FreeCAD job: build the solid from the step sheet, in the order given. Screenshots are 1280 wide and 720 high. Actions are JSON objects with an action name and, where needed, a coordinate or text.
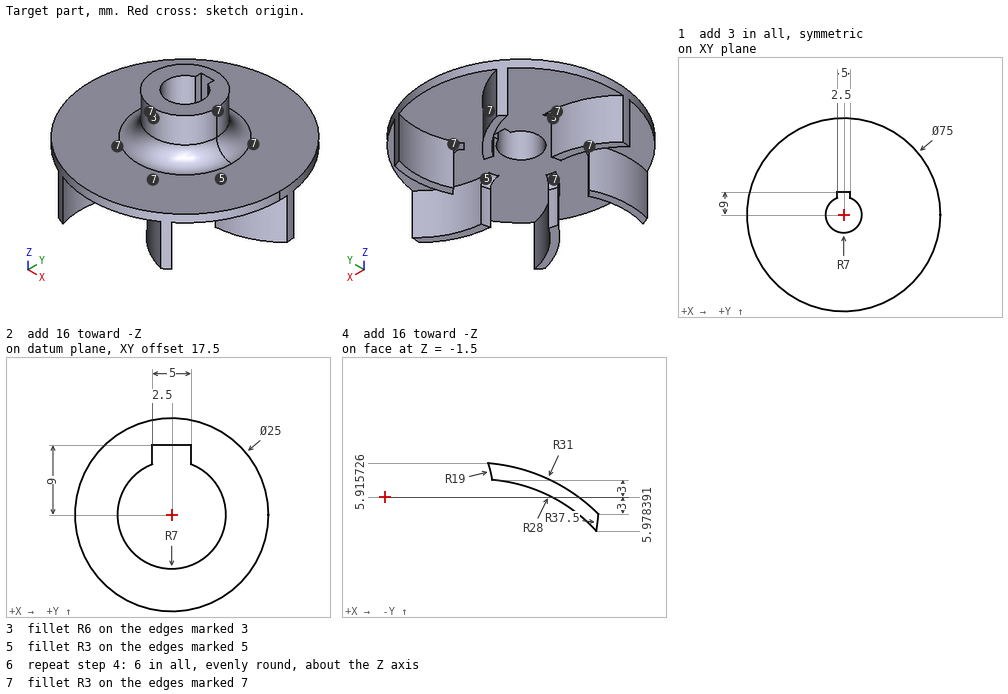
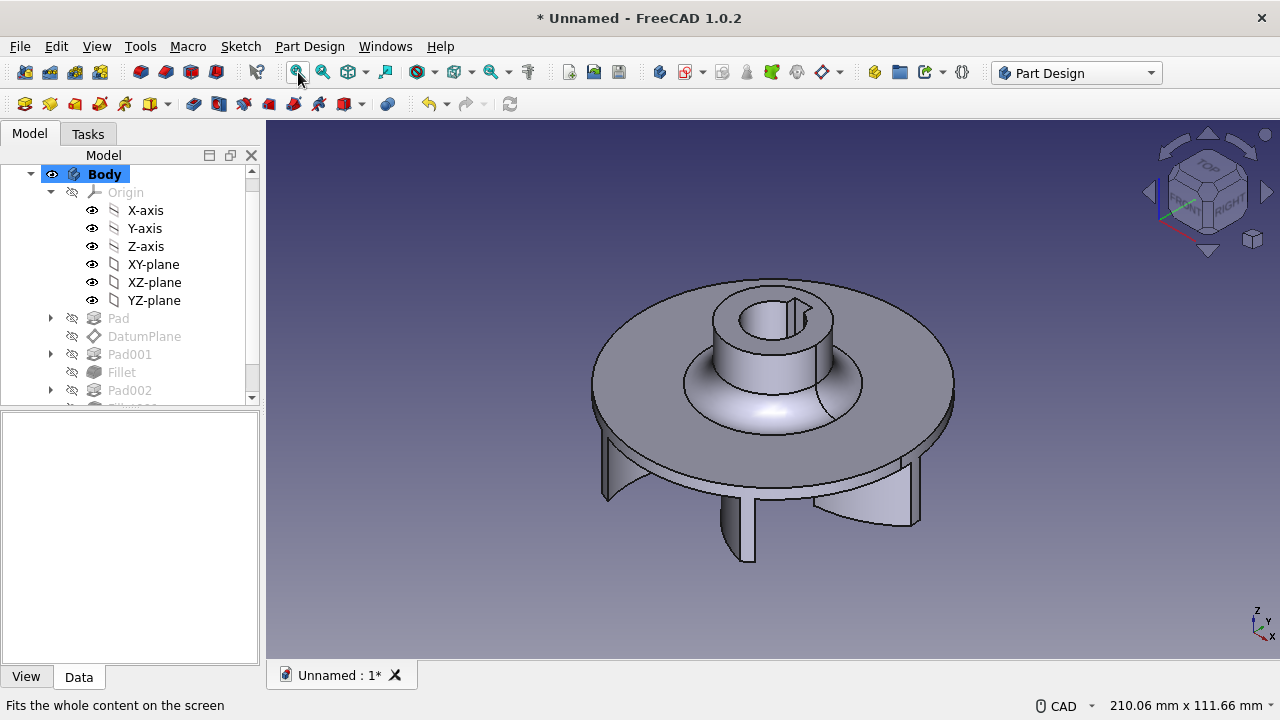
{"action": "scroll", "coordinate": [865, 393], "scroll_direction": "up", "scroll_amount": 6}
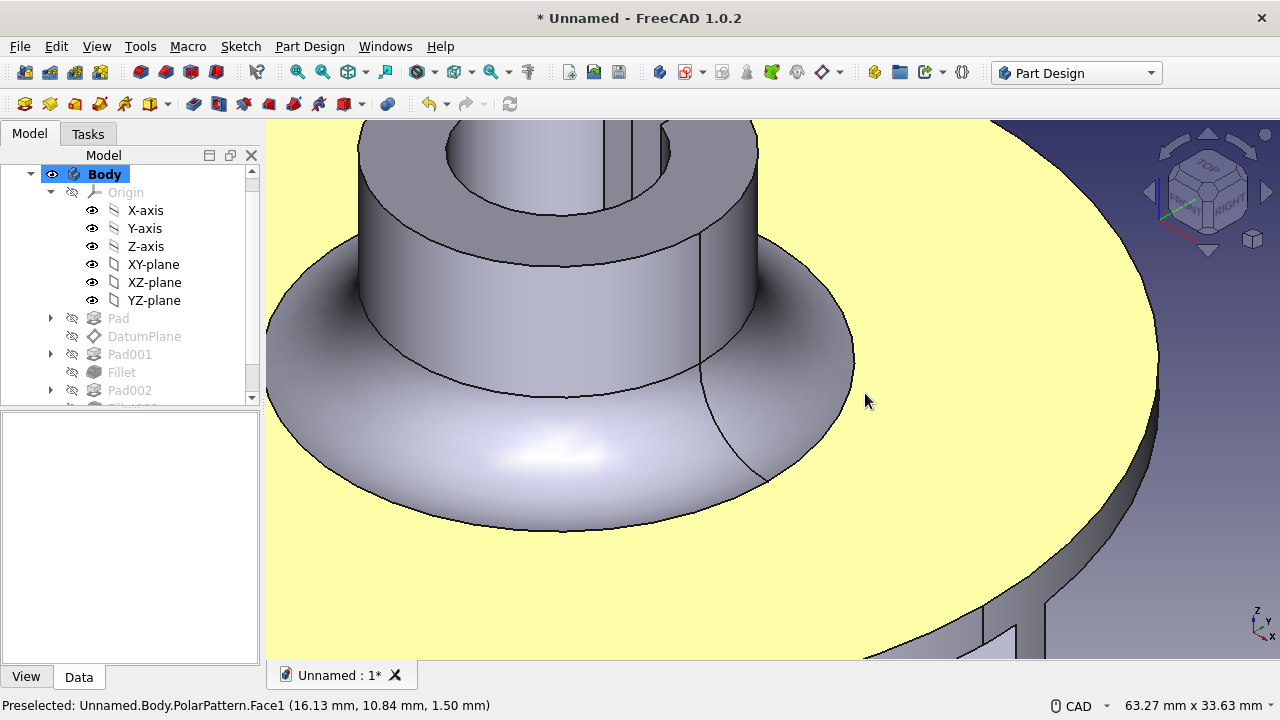
{"action": "key", "text": "v f"}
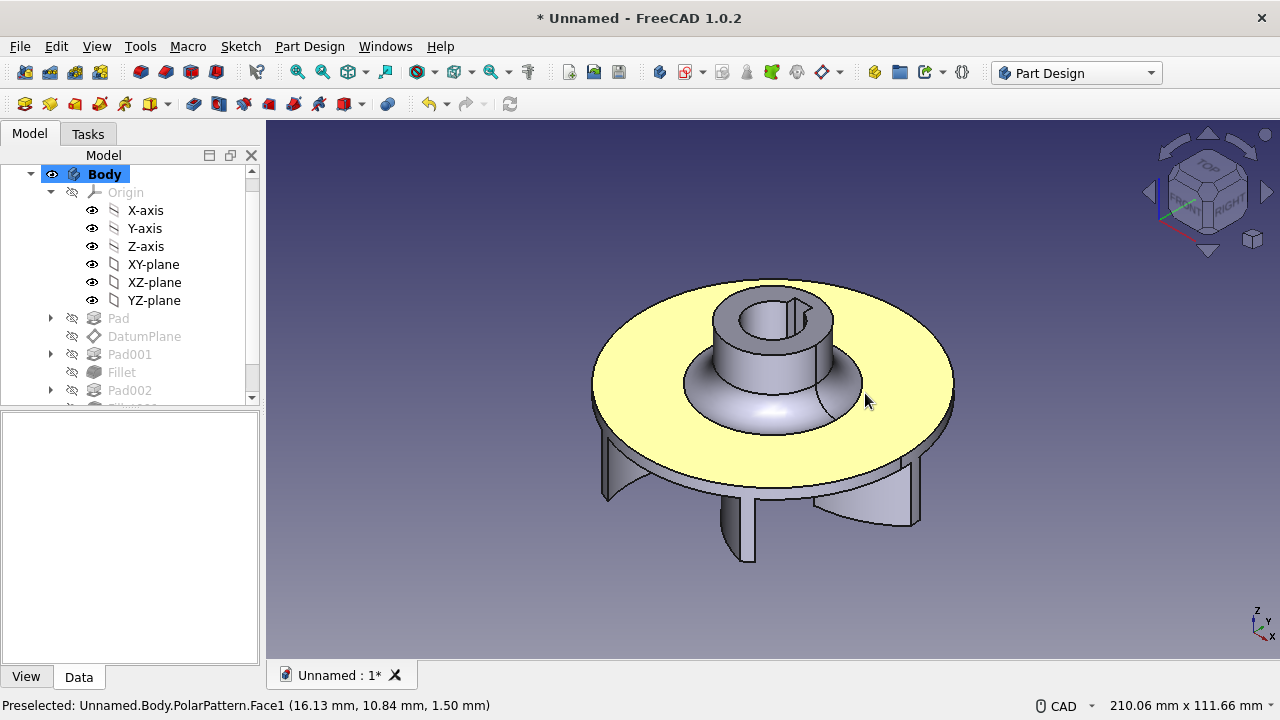
{"action": "key", "text": "1"}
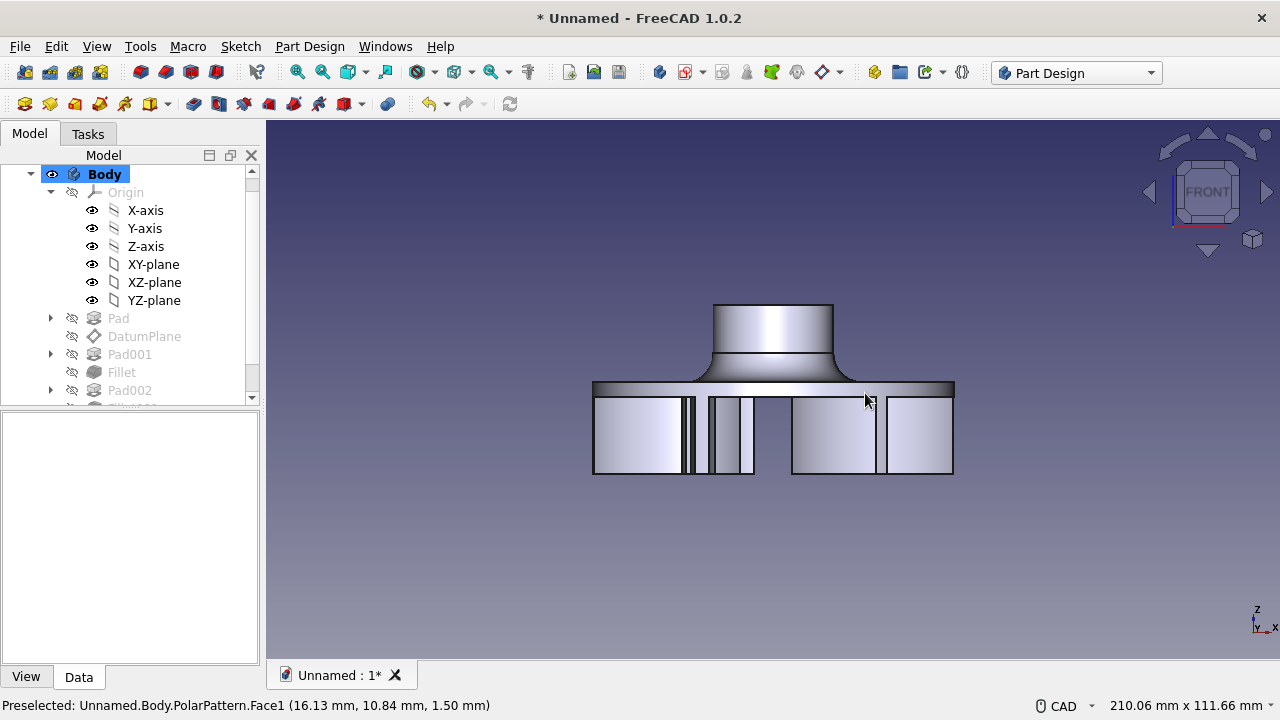
{"action": "left_click", "coordinate": [298, 72]}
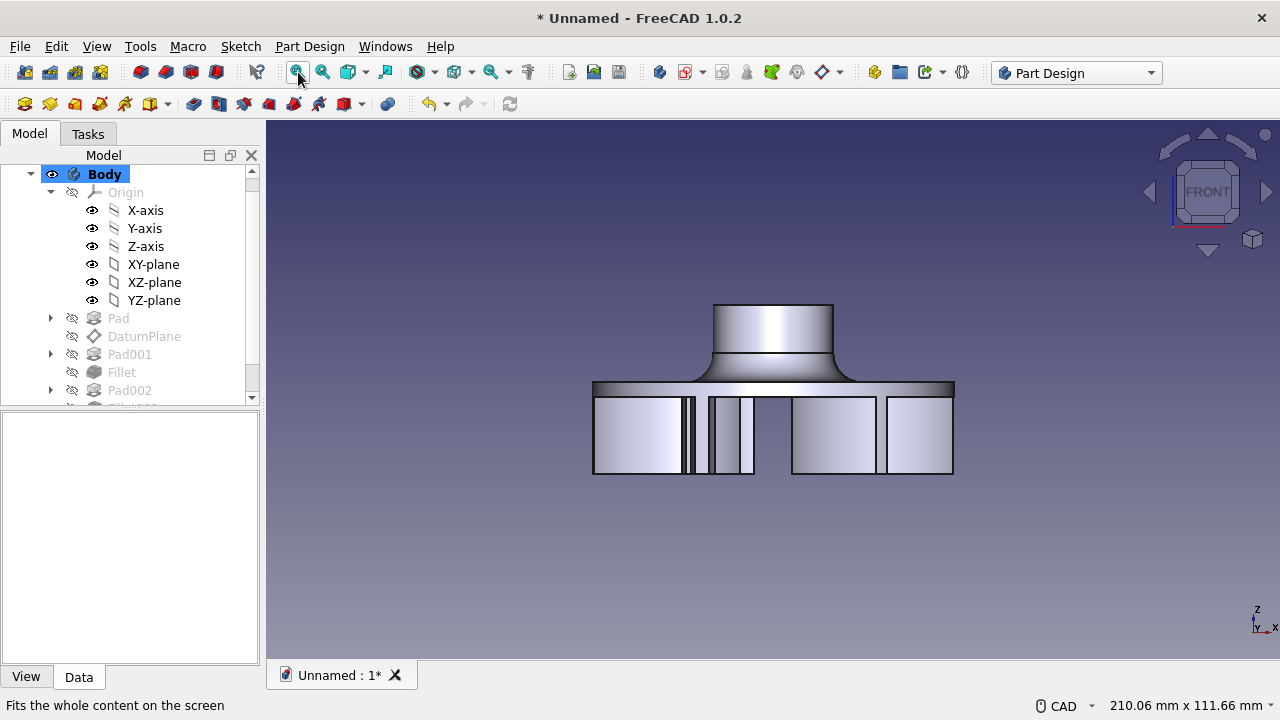
{"action": "scroll", "coordinate": [836, 396], "scroll_direction": "up", "scroll_amount": 6}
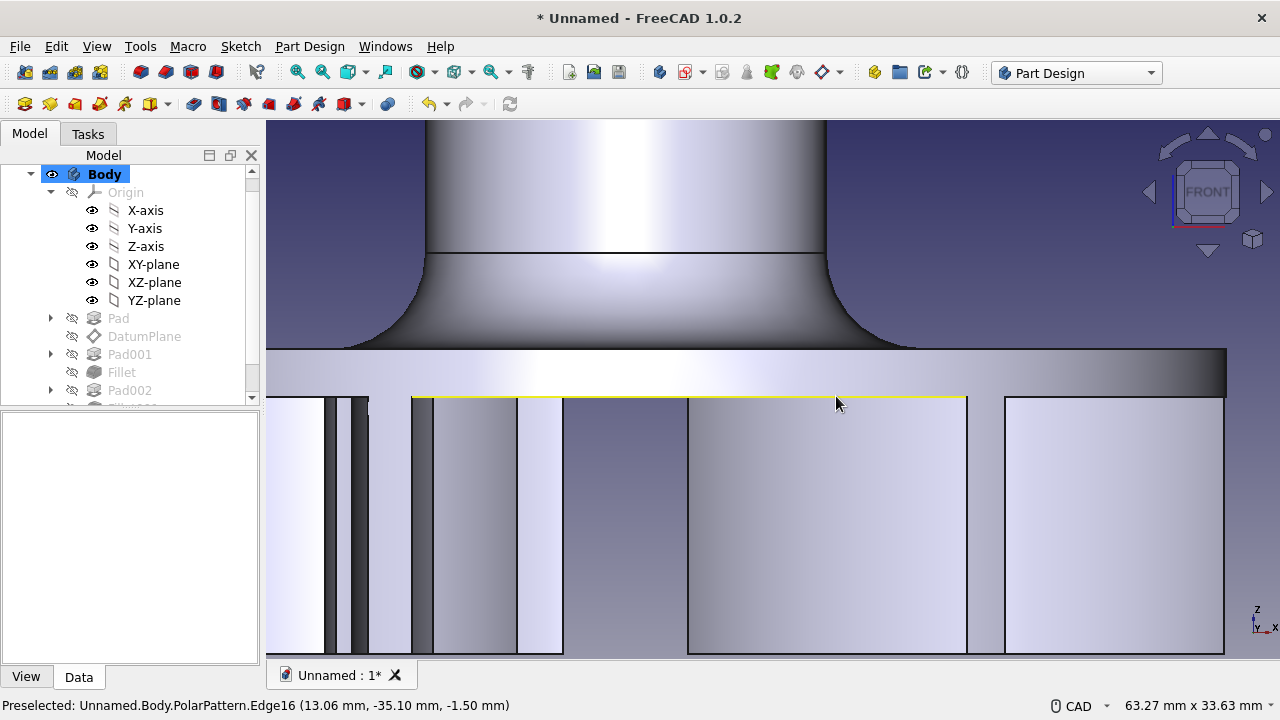
{"action": "key", "text": "v f"}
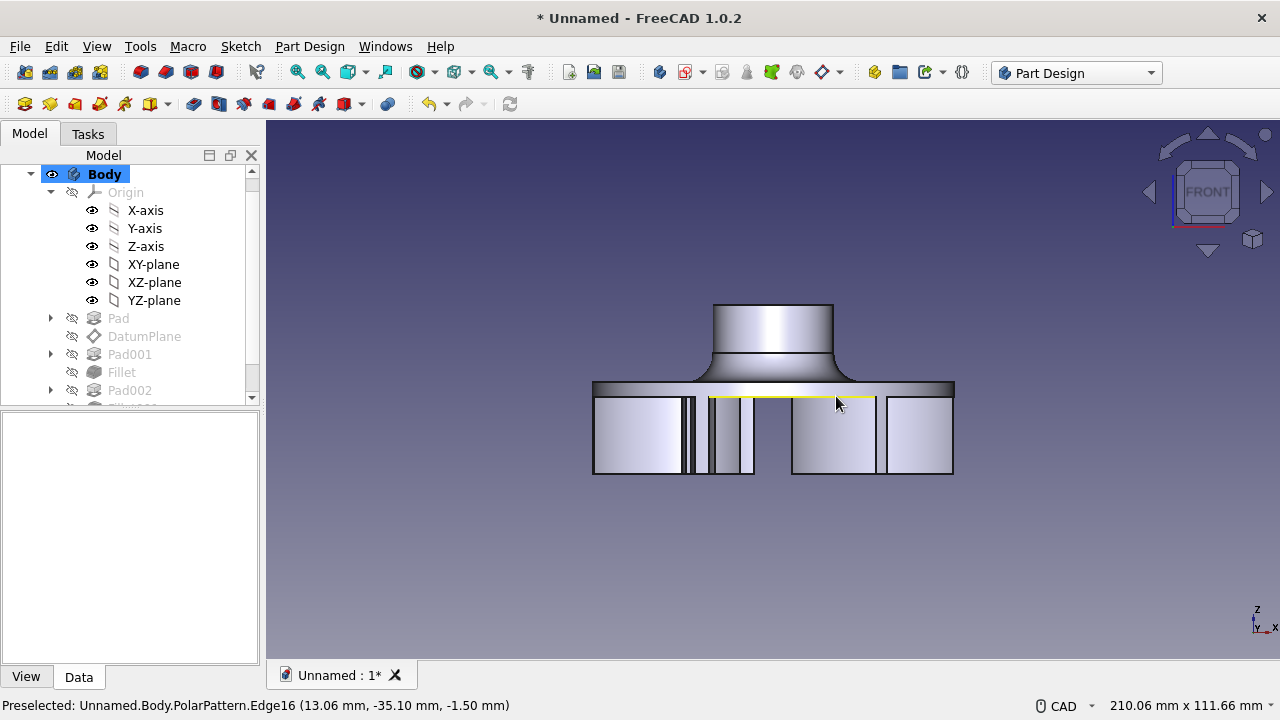
{"action": "key", "text": "3"}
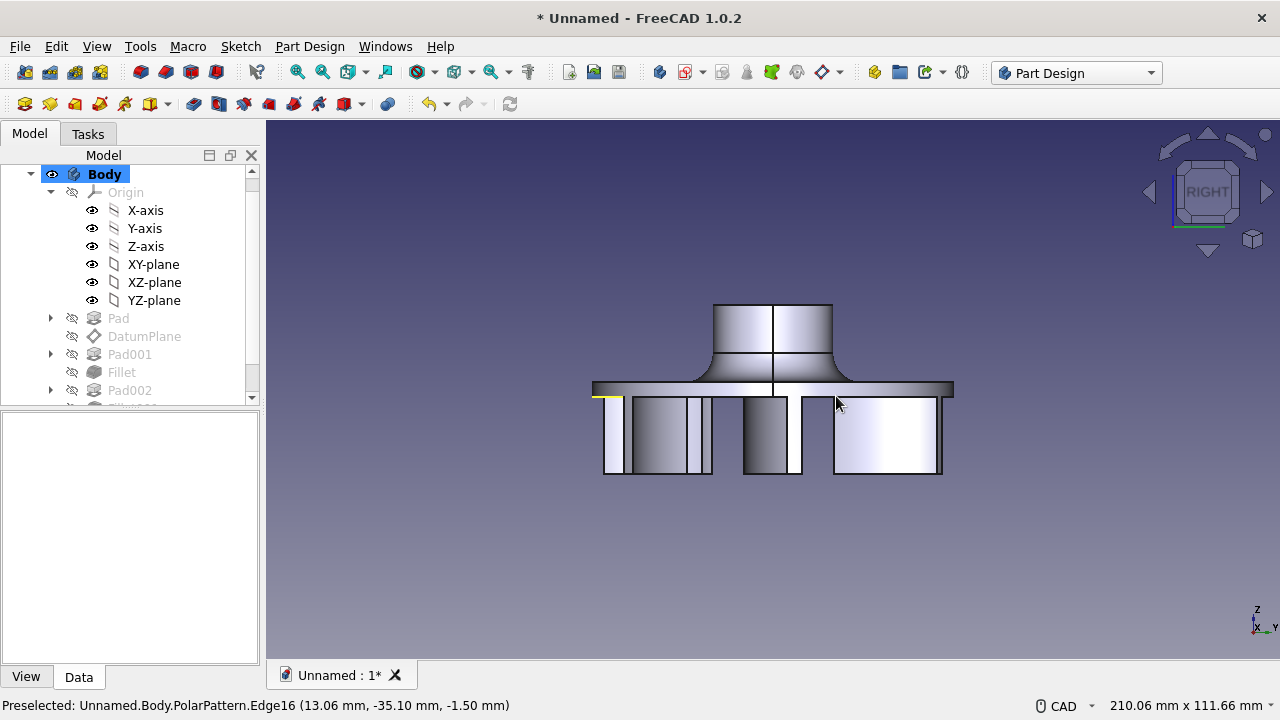
{"action": "left_click", "coordinate": [298, 72]}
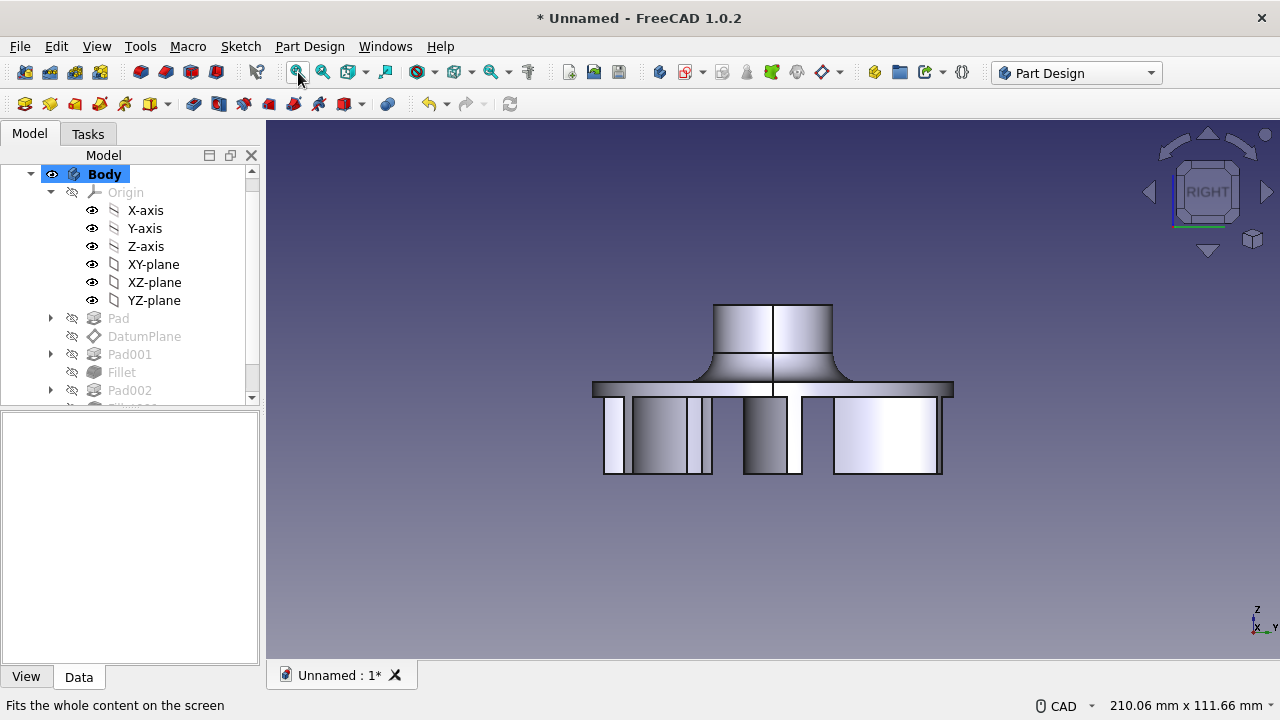
{"action": "scroll", "coordinate": [839, 396], "scroll_direction": "up", "scroll_amount": 6}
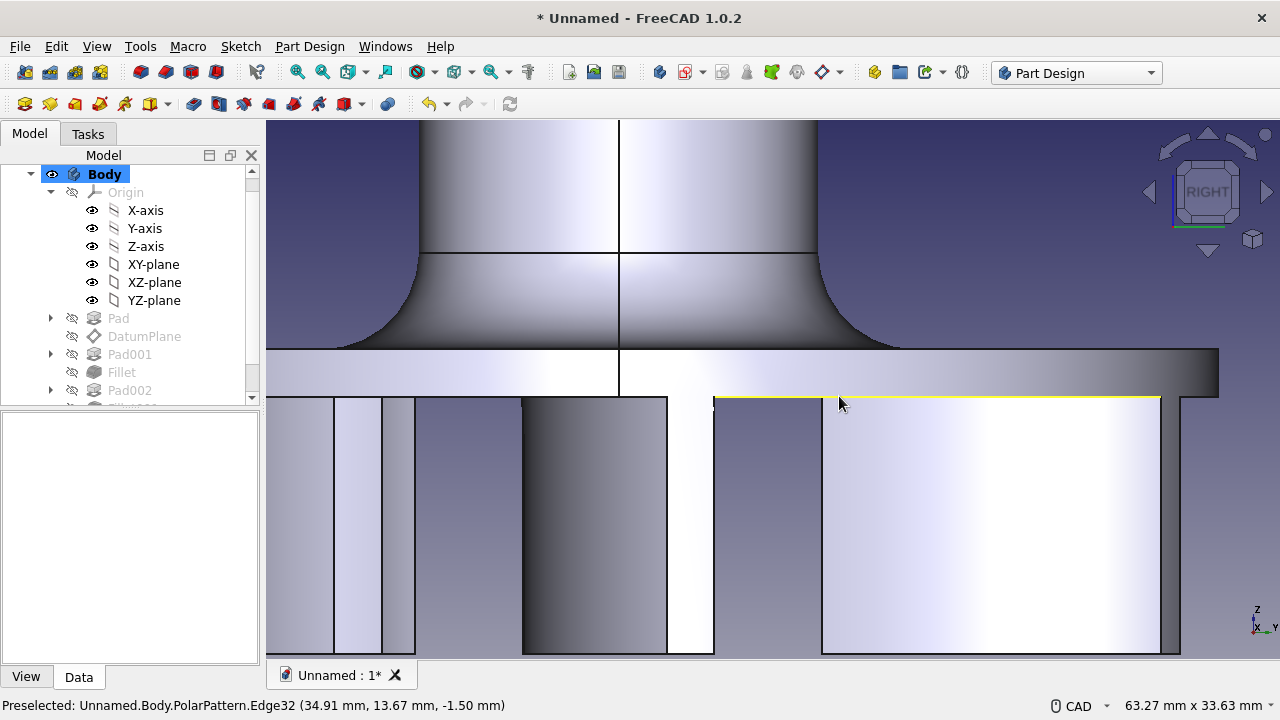
{"action": "left_click", "coordinate": [298, 72]}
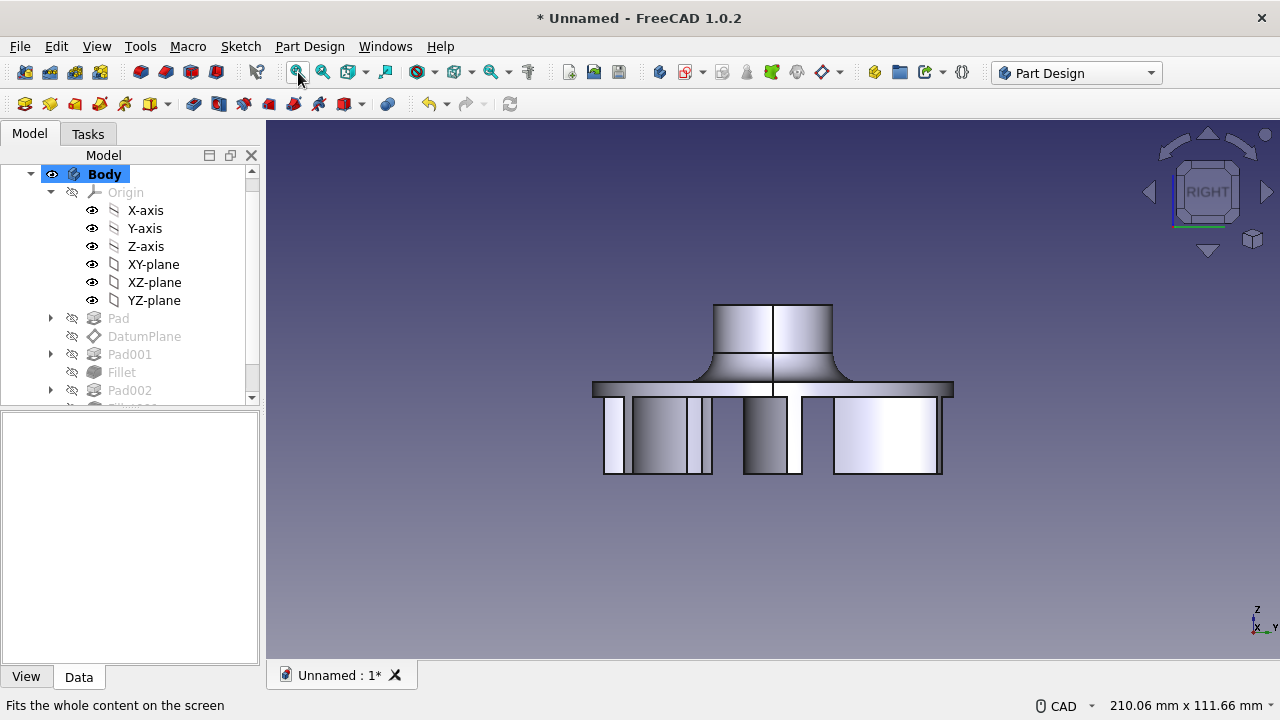
{"action": "key", "text": "5"}